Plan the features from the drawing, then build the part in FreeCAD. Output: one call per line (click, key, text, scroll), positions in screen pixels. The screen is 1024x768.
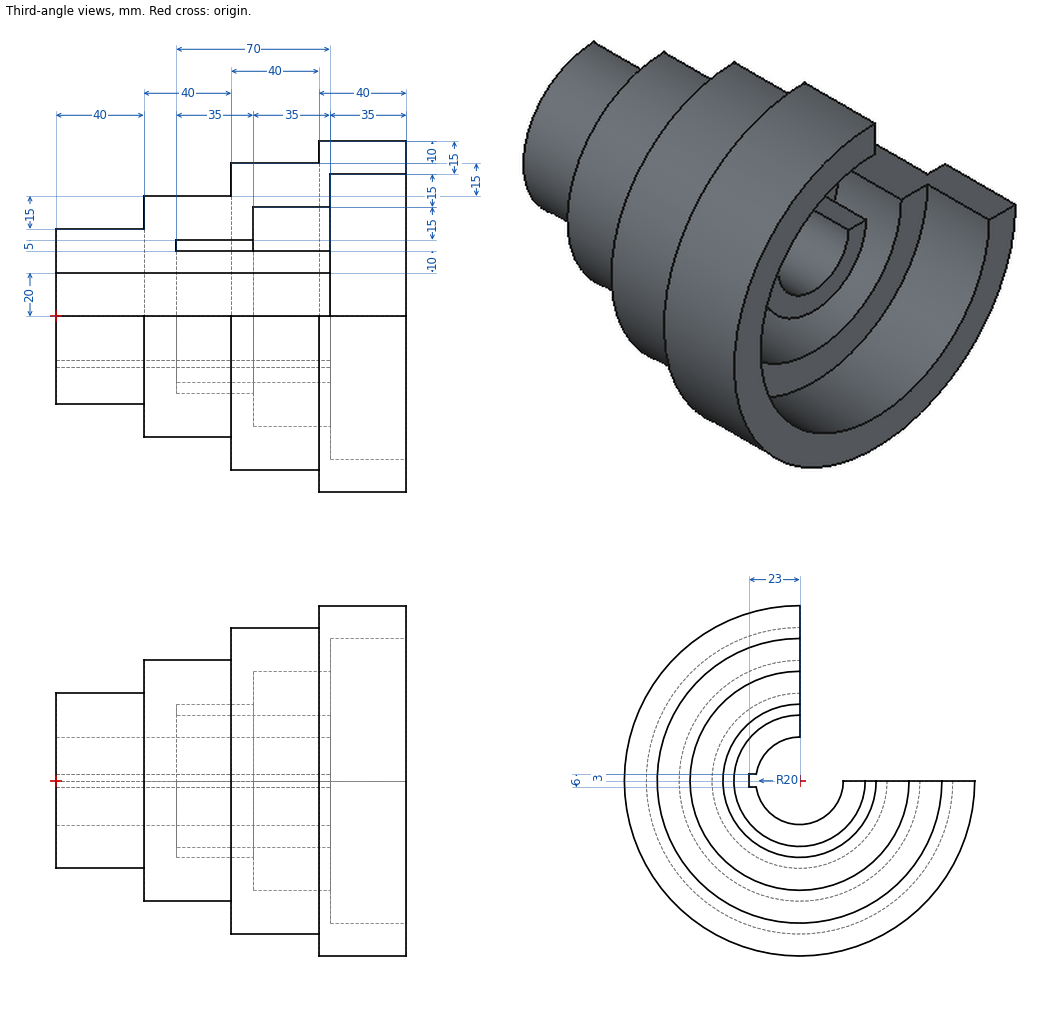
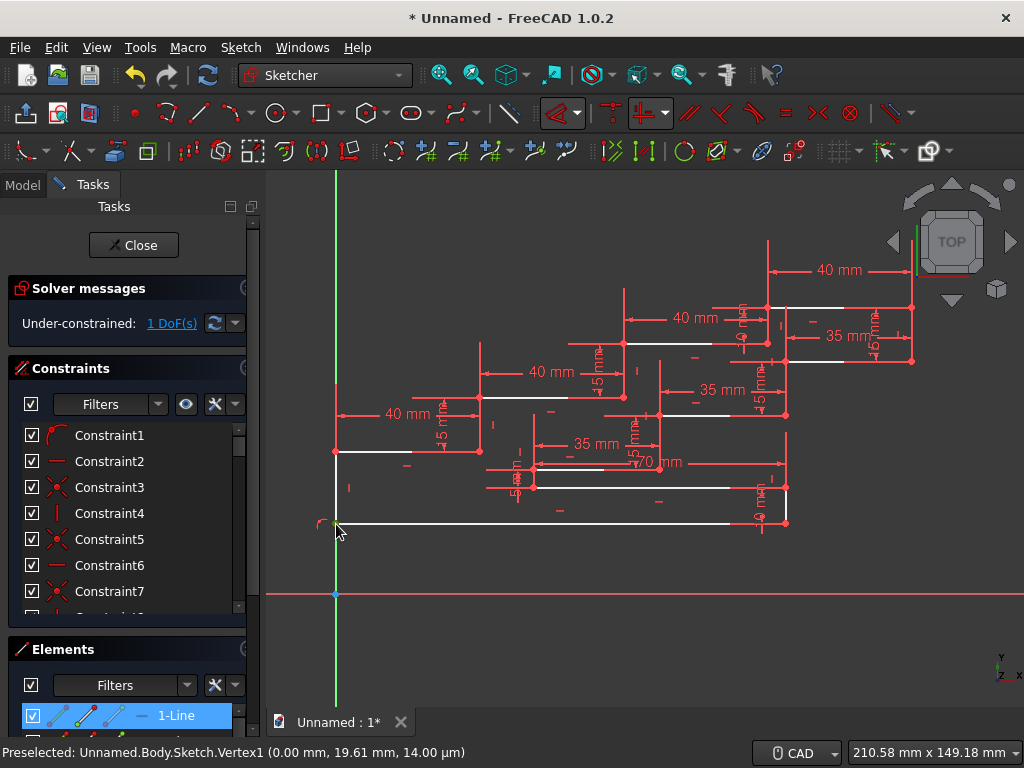
key(i)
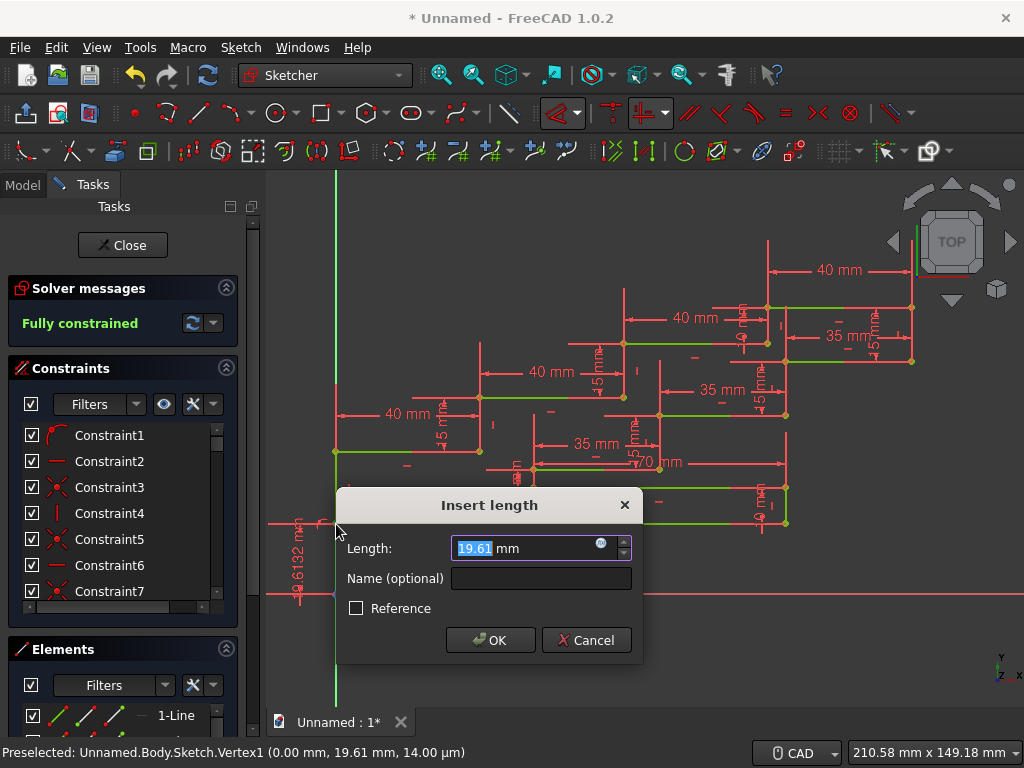
text(20)
key(Return)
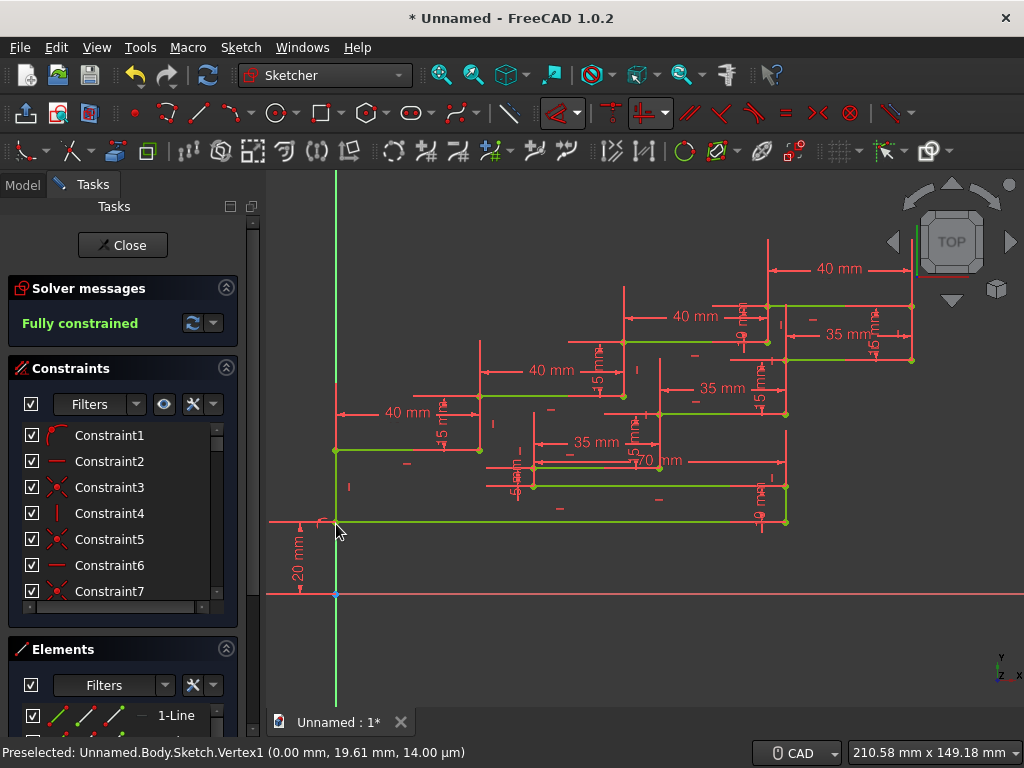
click(123, 245)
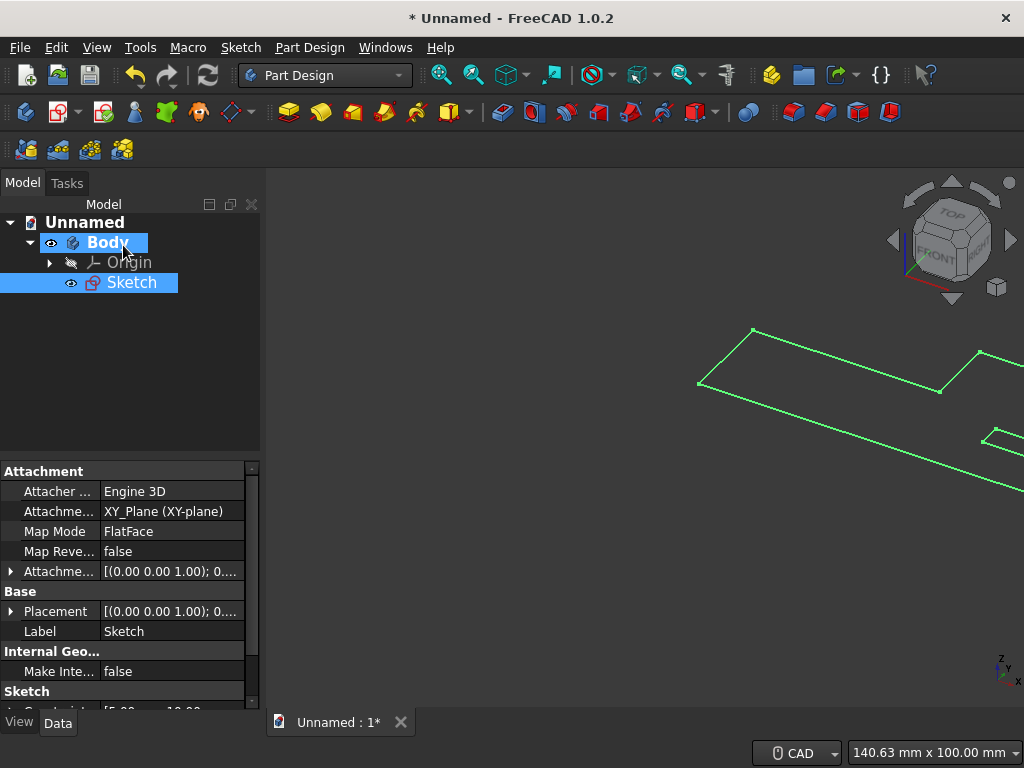
click(322, 112)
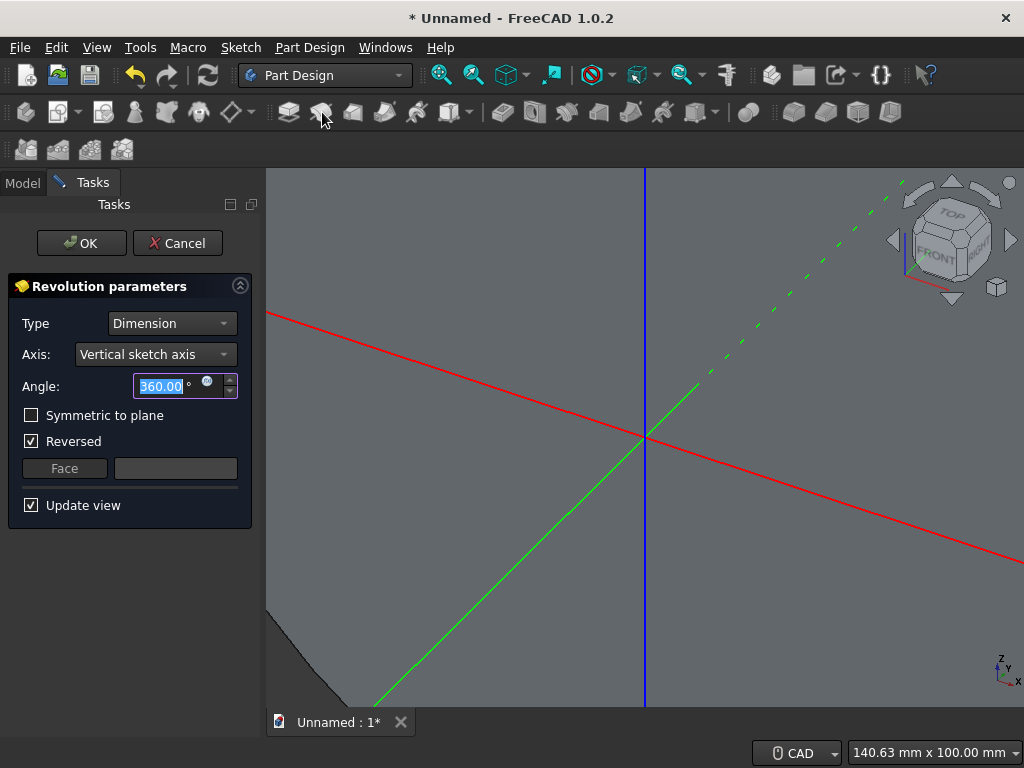
click(156, 354)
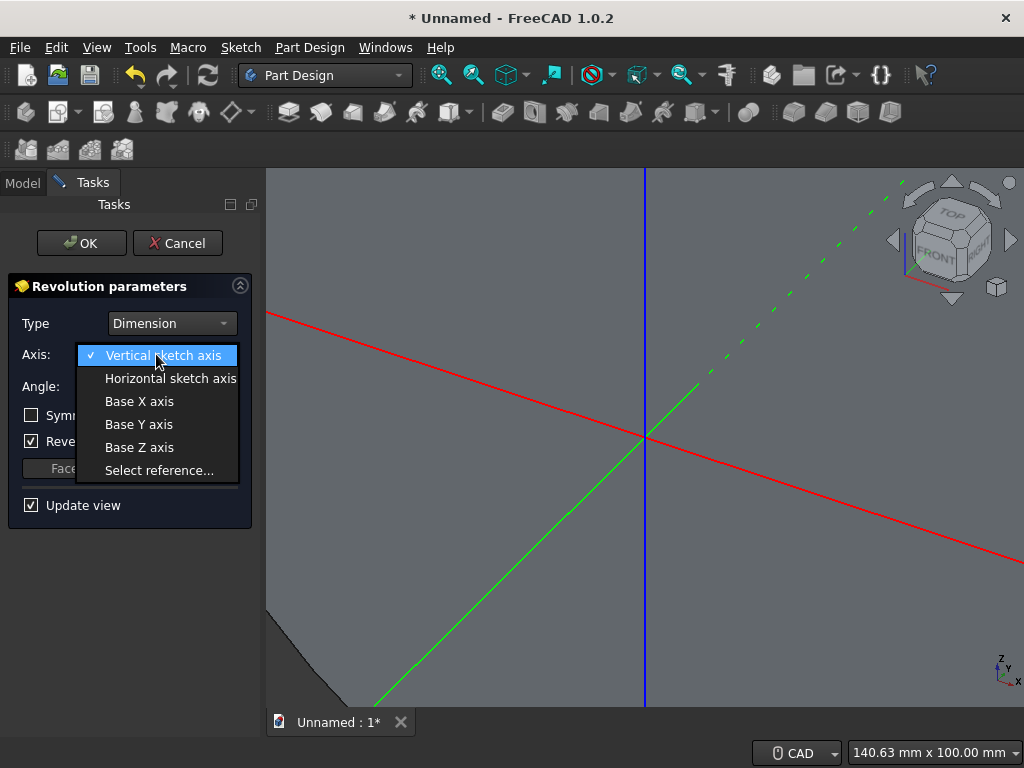
click(156, 378)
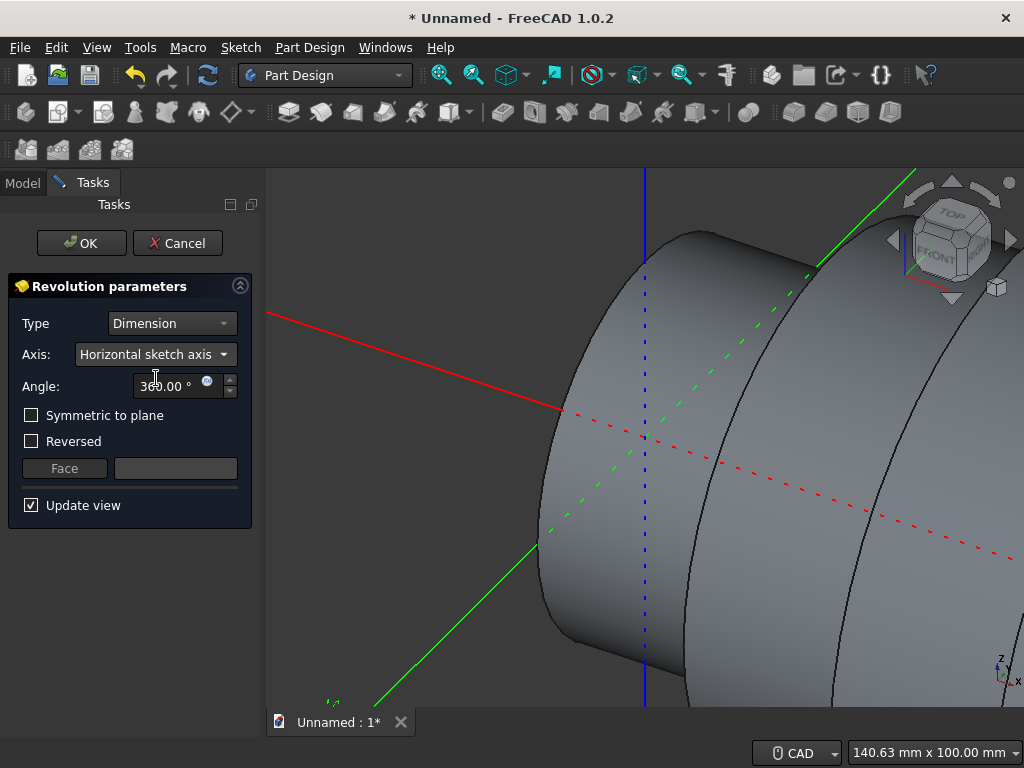
triple_click(178, 386)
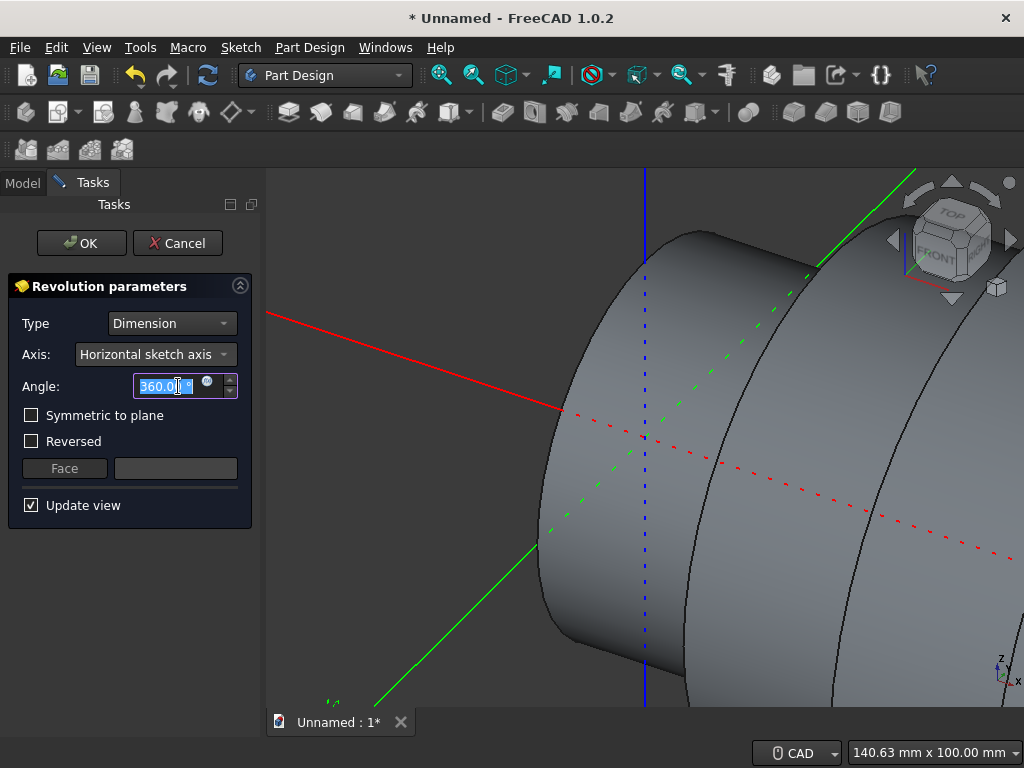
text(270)
key(Tab)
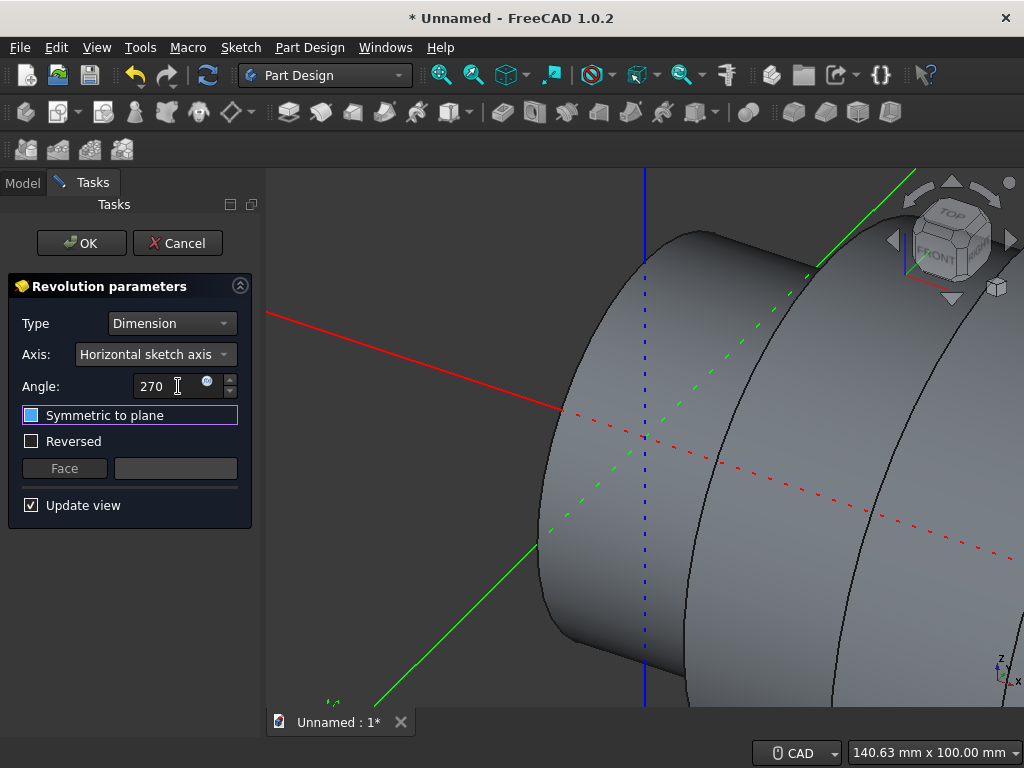
click(30, 441)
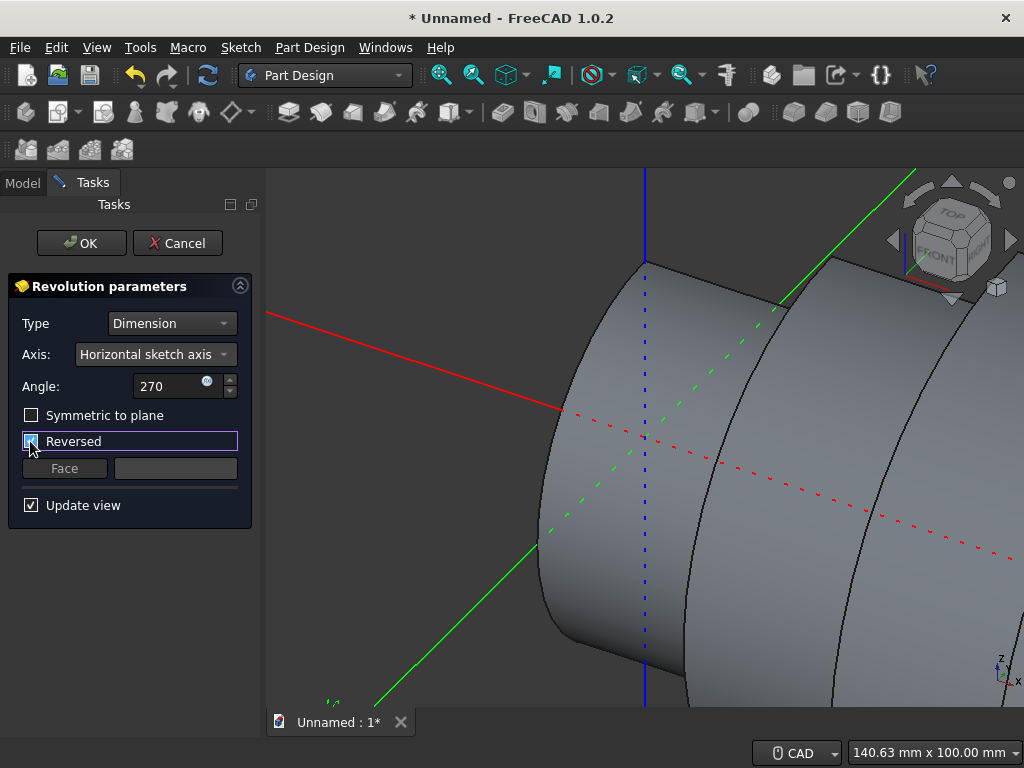
click(82, 243)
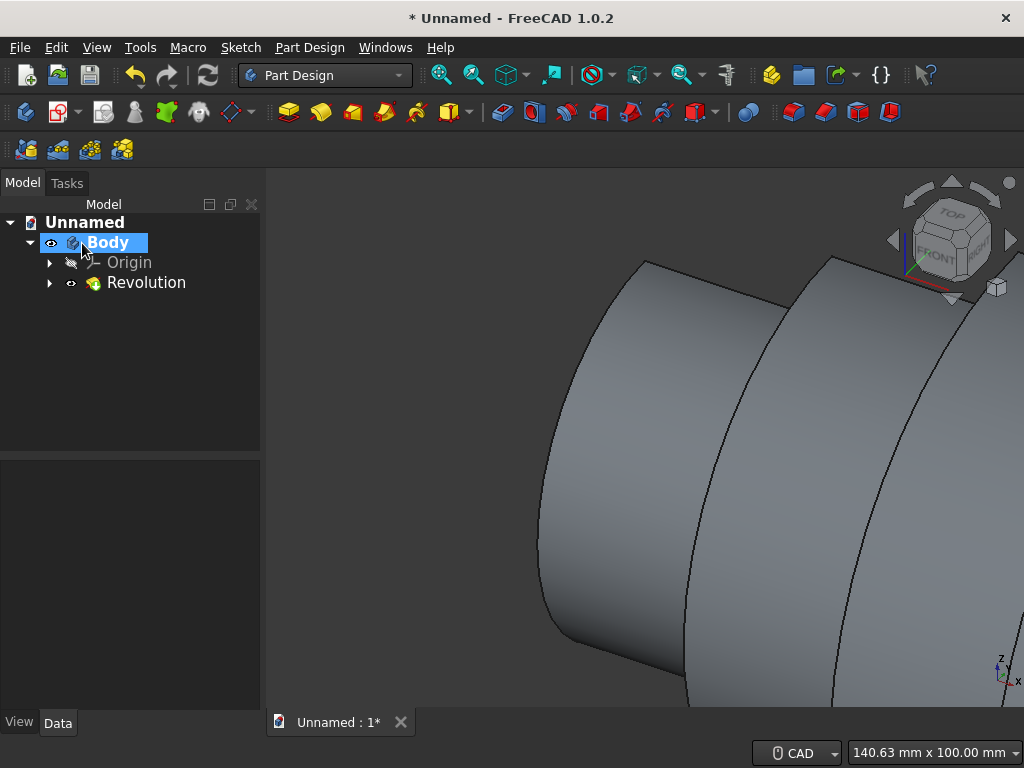
click(442, 76)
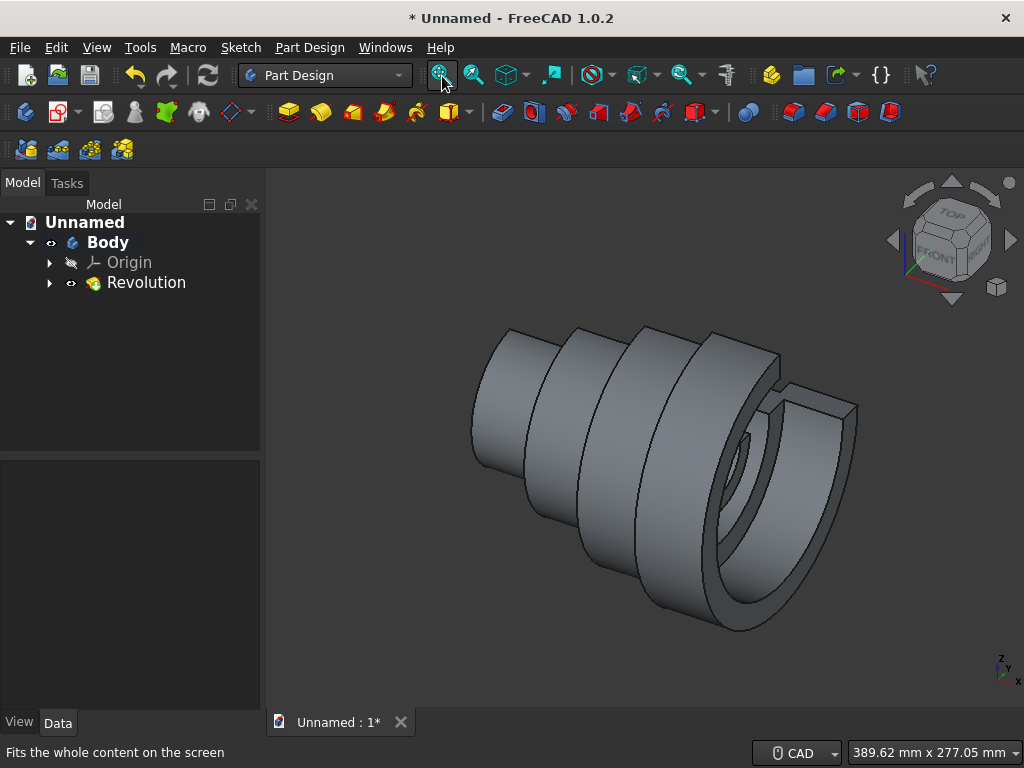
key(6)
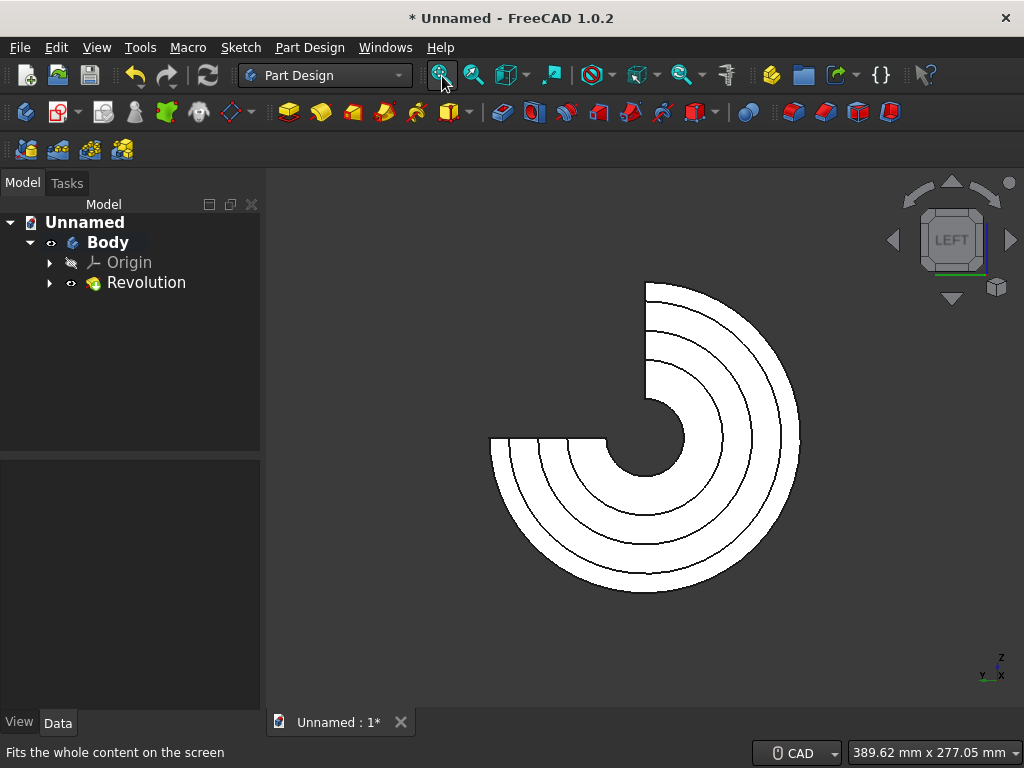
click(601, 481)